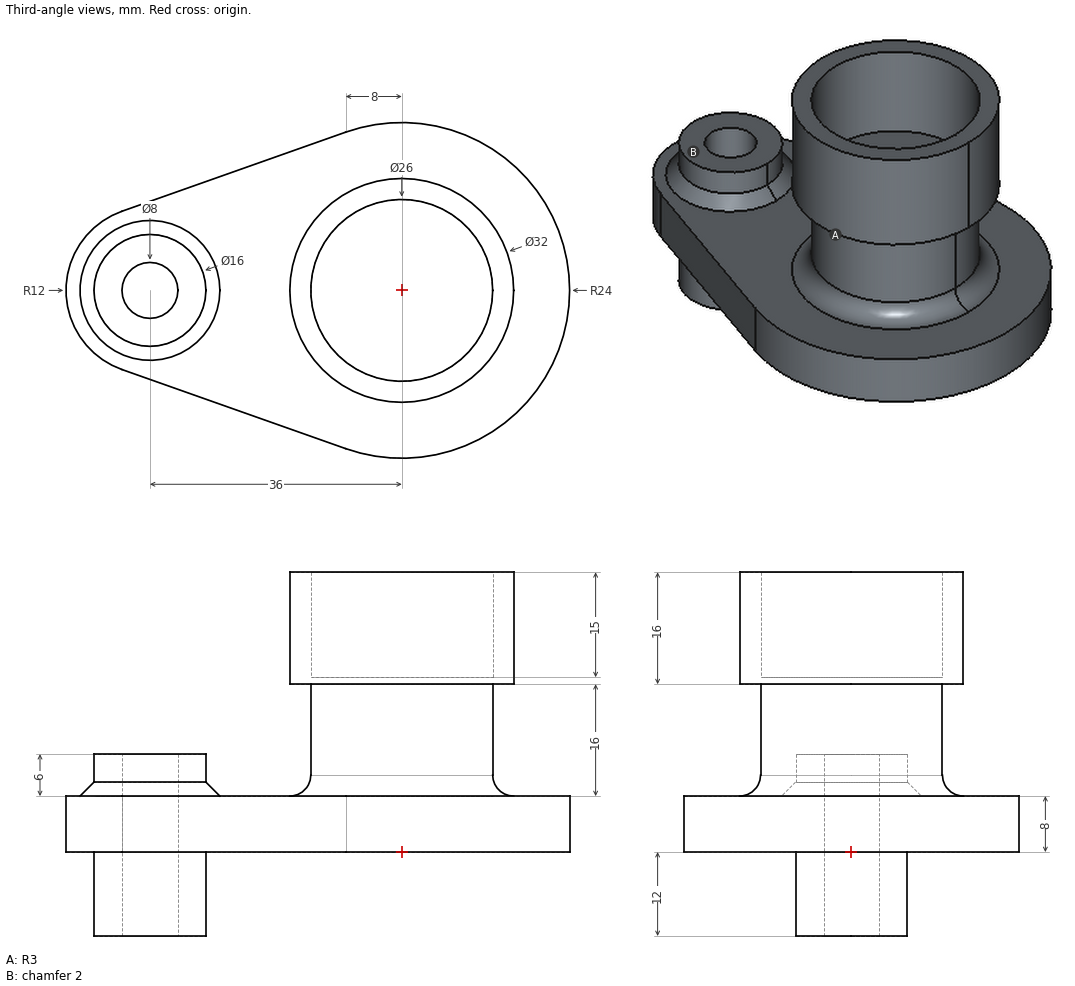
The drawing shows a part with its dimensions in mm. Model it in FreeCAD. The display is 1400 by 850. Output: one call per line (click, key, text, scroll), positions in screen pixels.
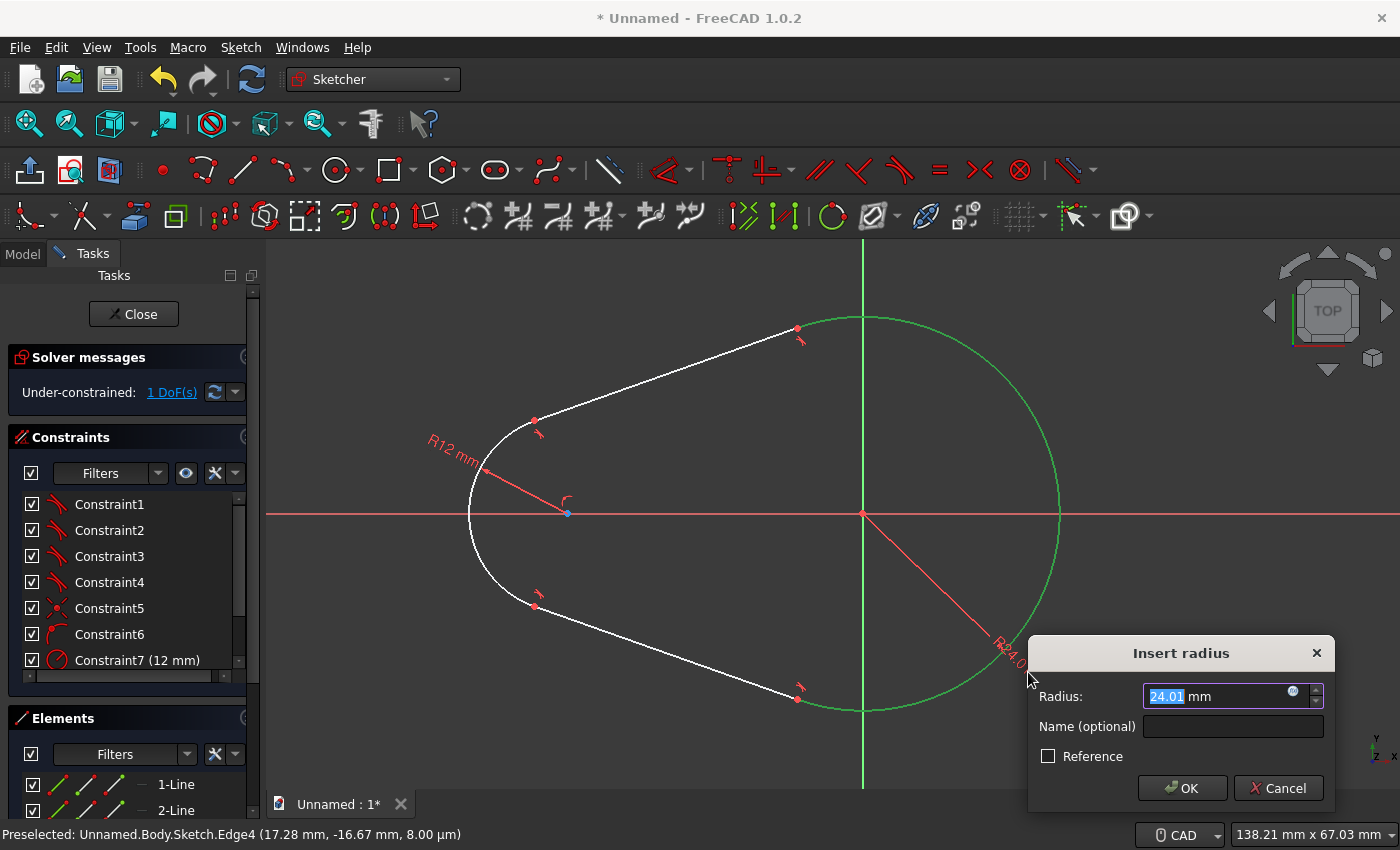
text(24)
key(Return)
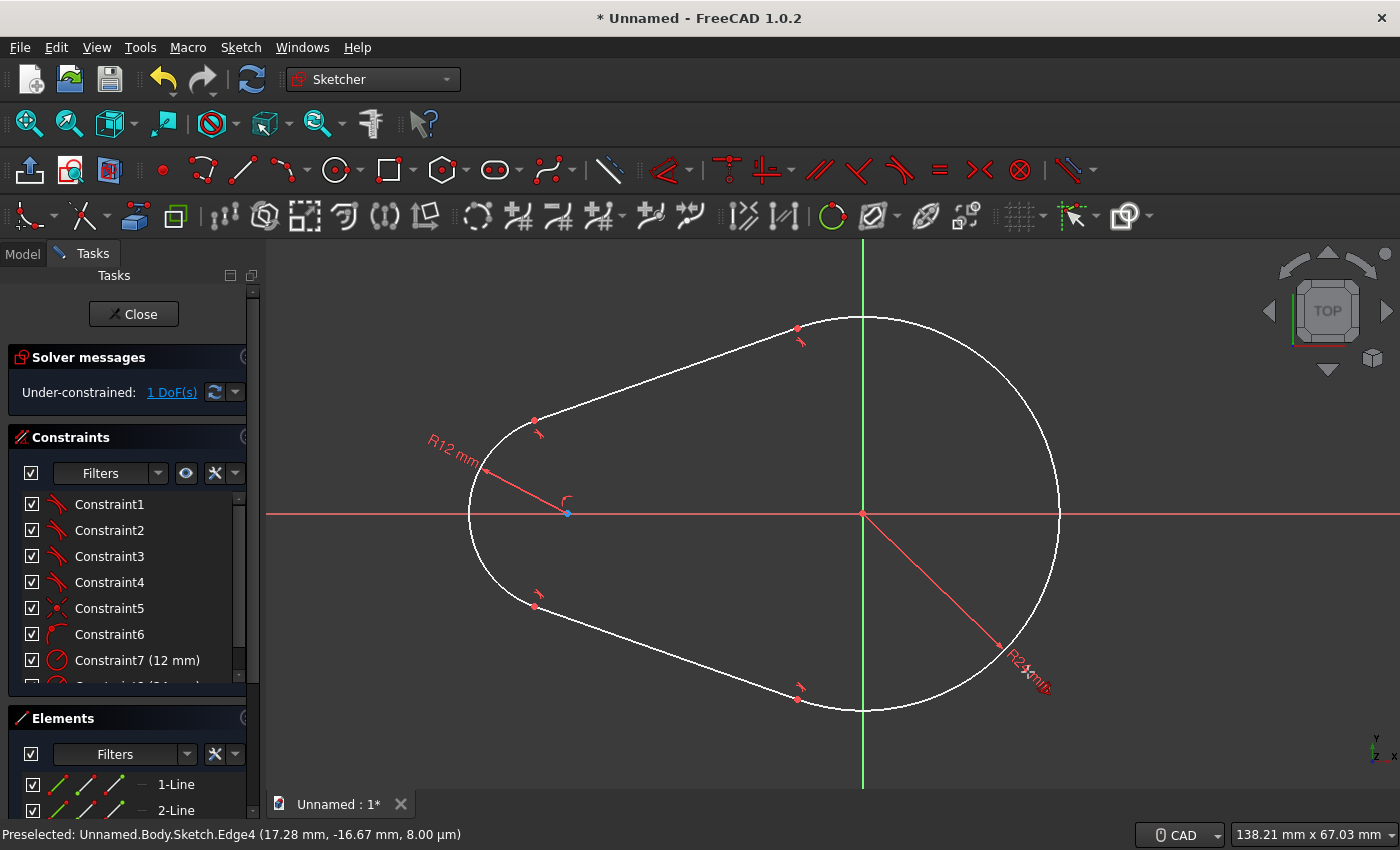
click(797, 328)
click(830, 294)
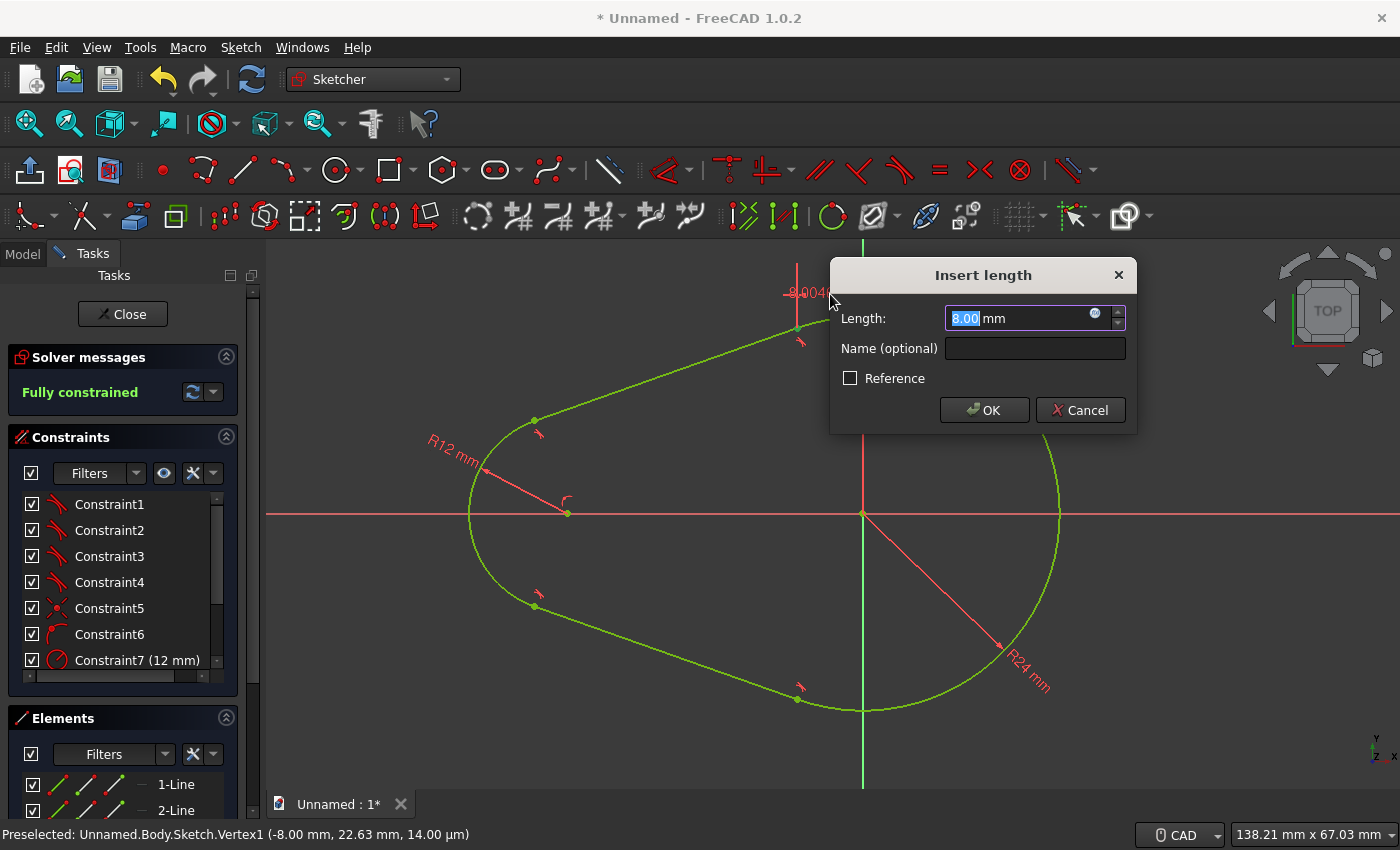
text(8)
key(Return)
key(Escape)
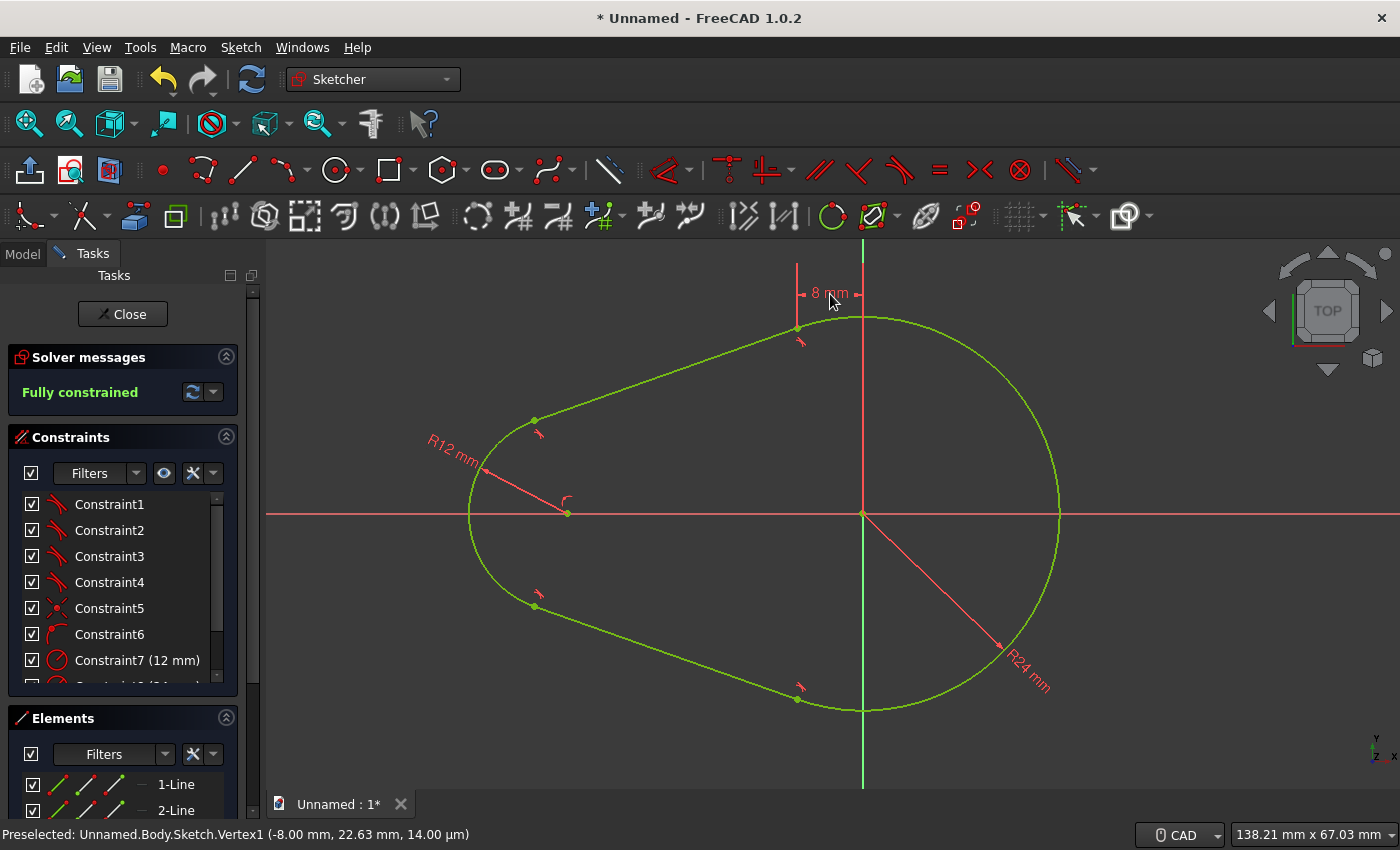
click(123, 314)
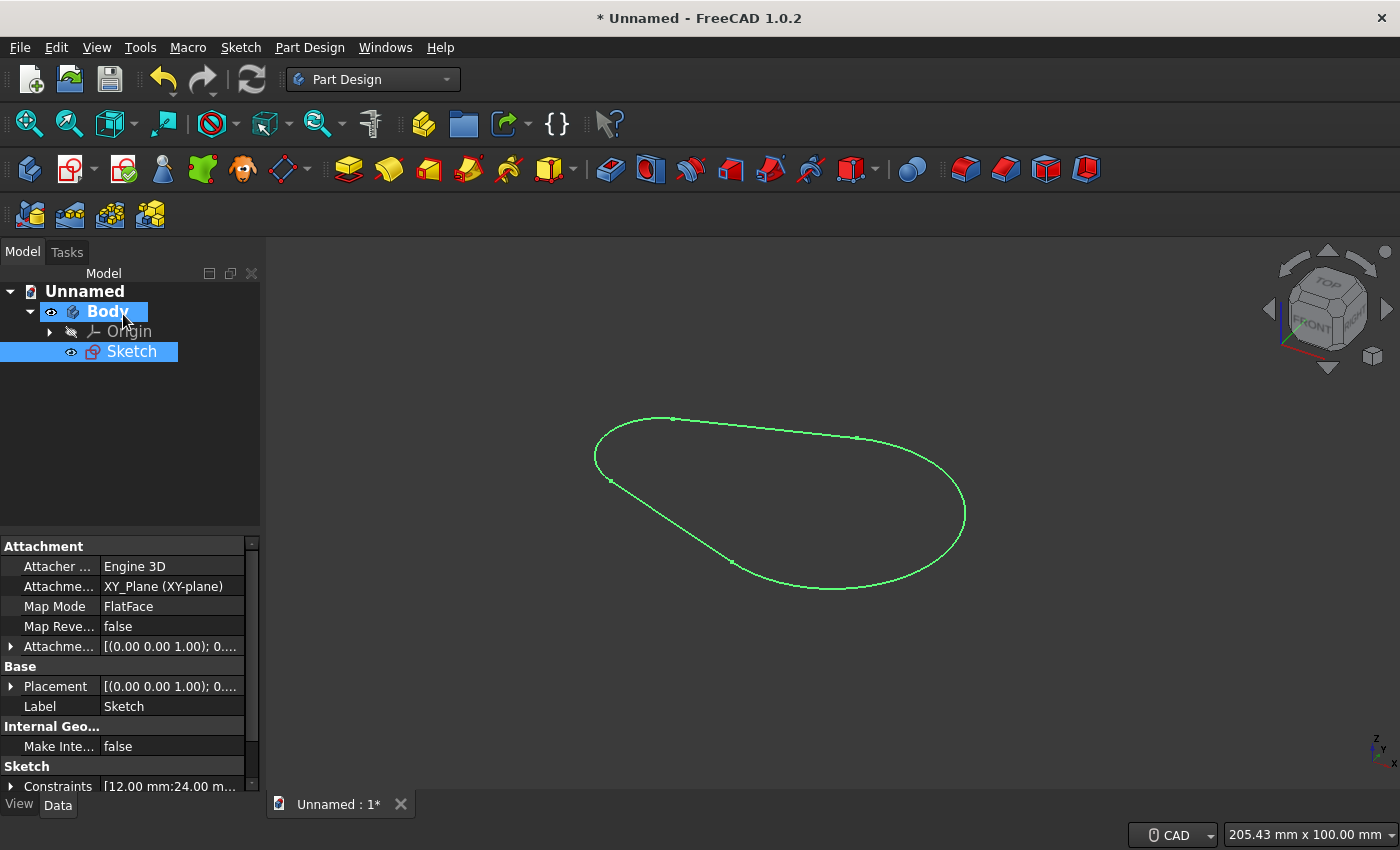
click(350, 170)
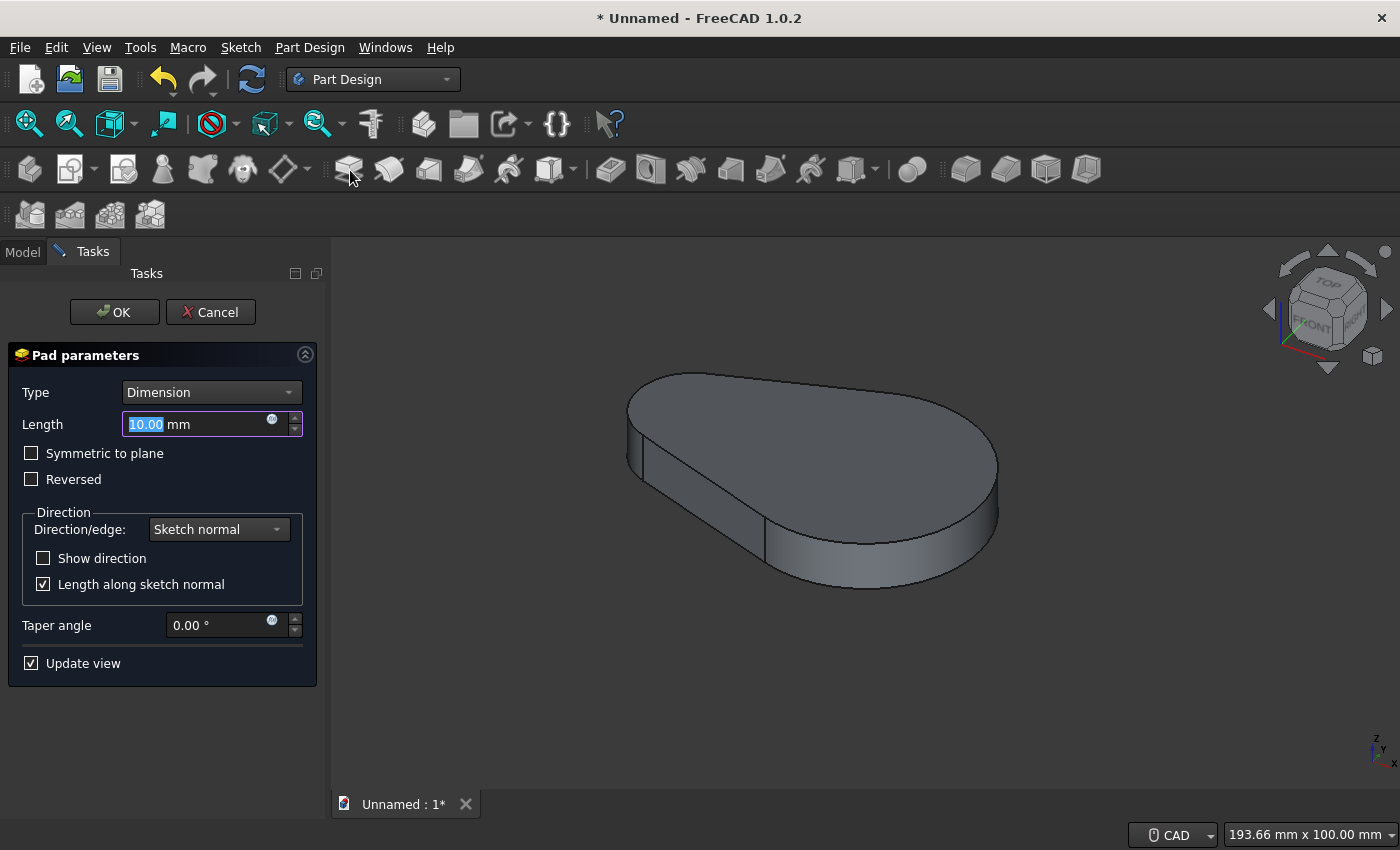
text(8)
key(Tab)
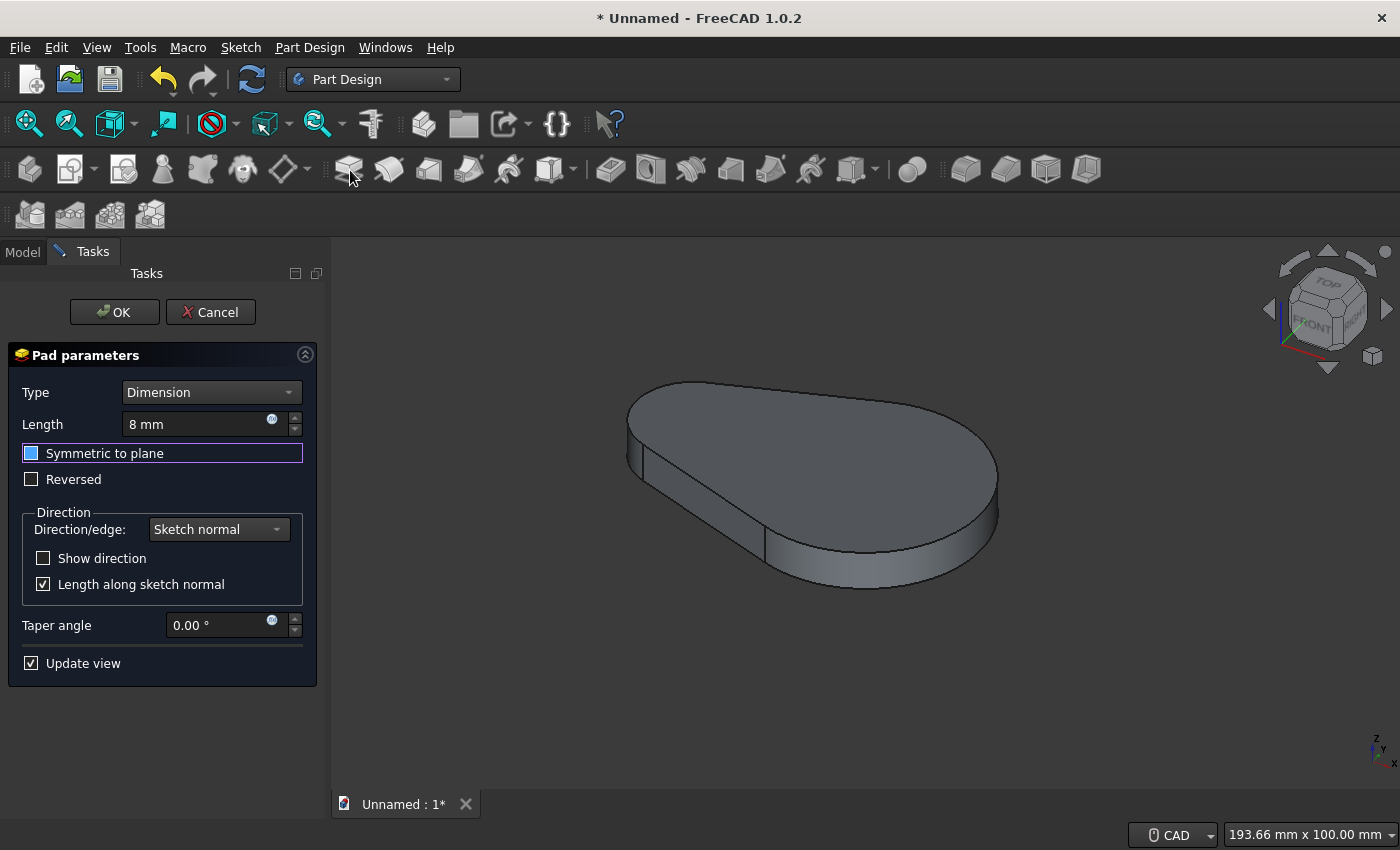
click(115, 312)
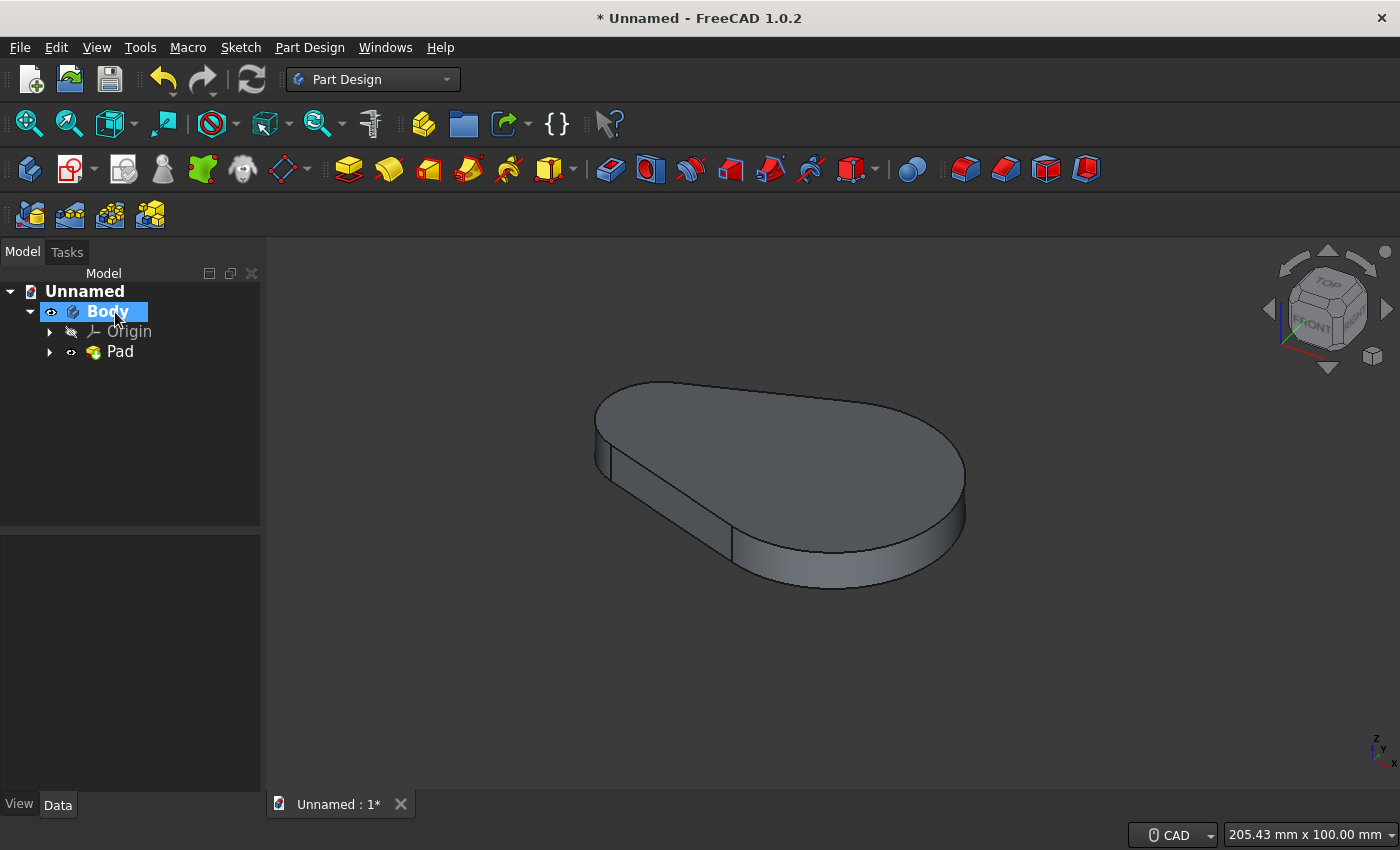
click(825, 473)